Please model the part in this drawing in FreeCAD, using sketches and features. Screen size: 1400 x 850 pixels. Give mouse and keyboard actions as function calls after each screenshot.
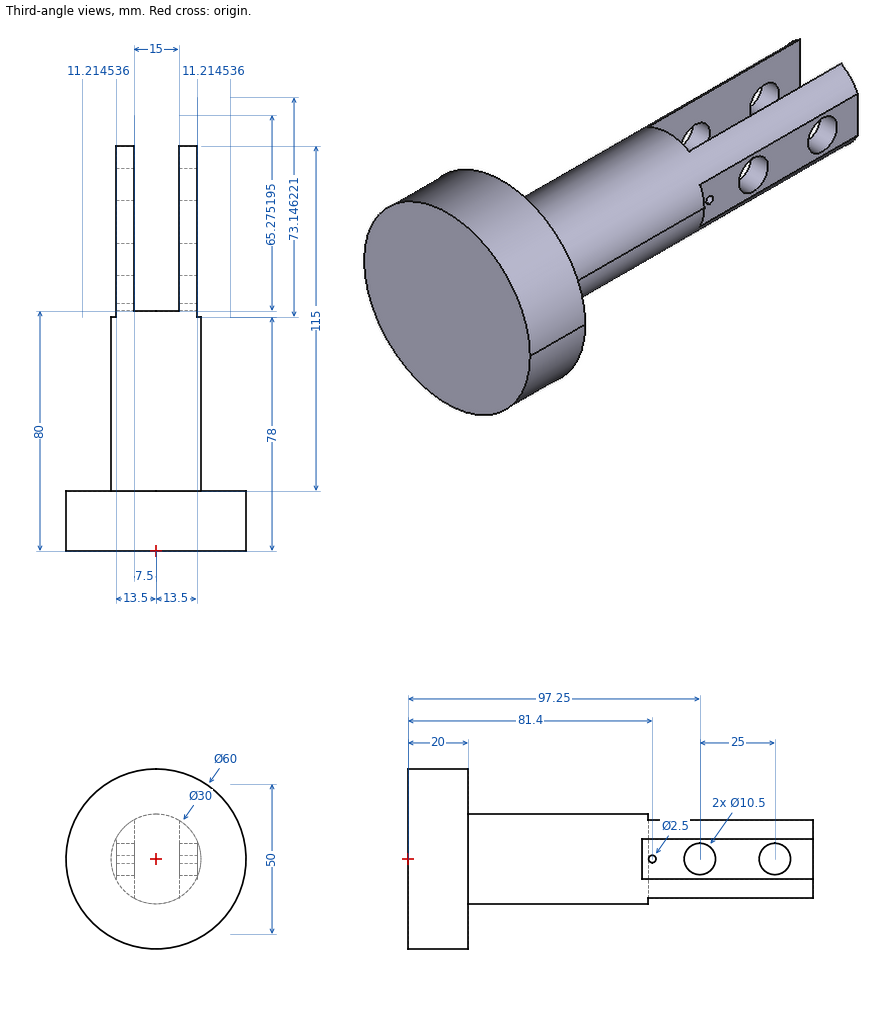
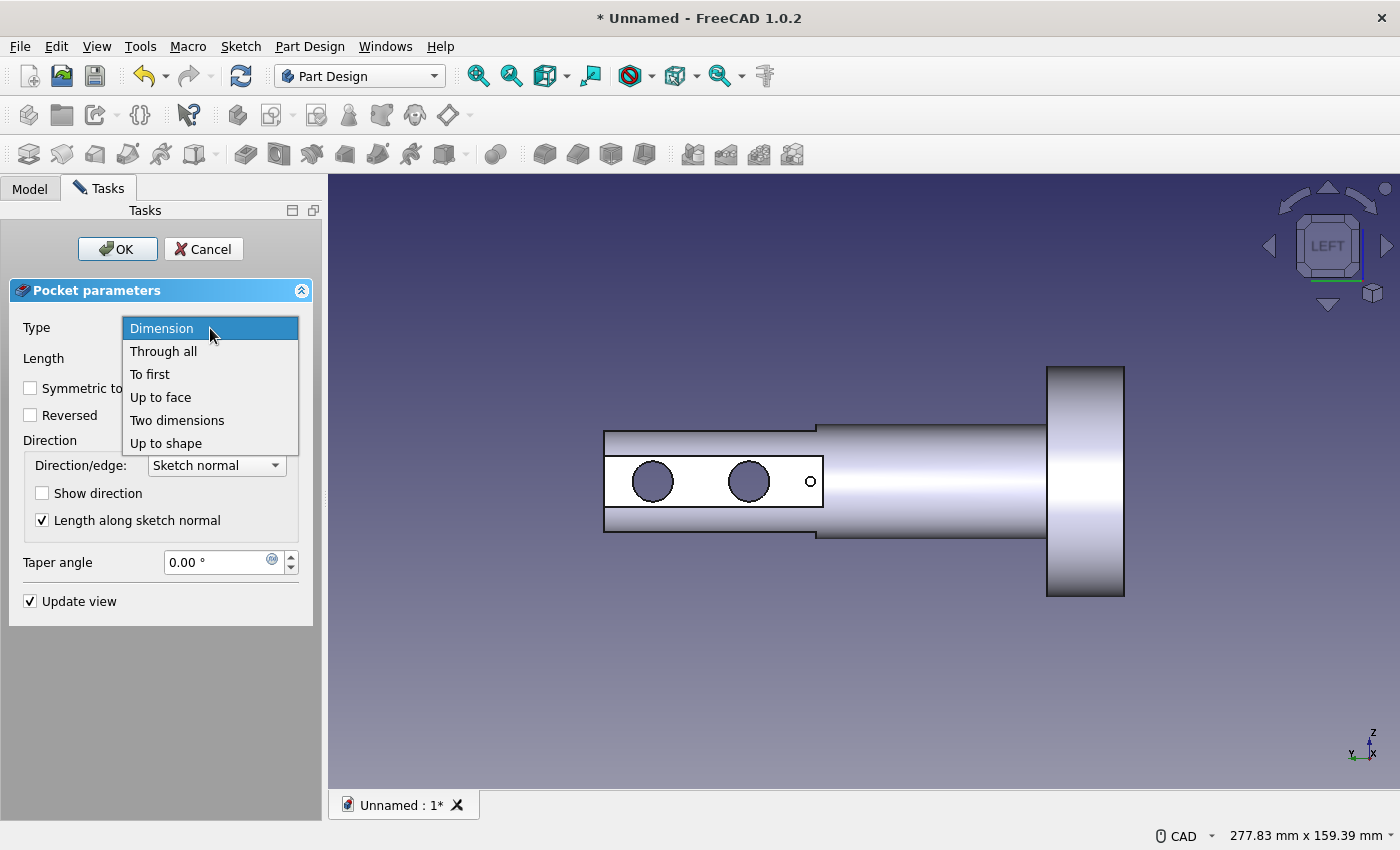
click(208, 352)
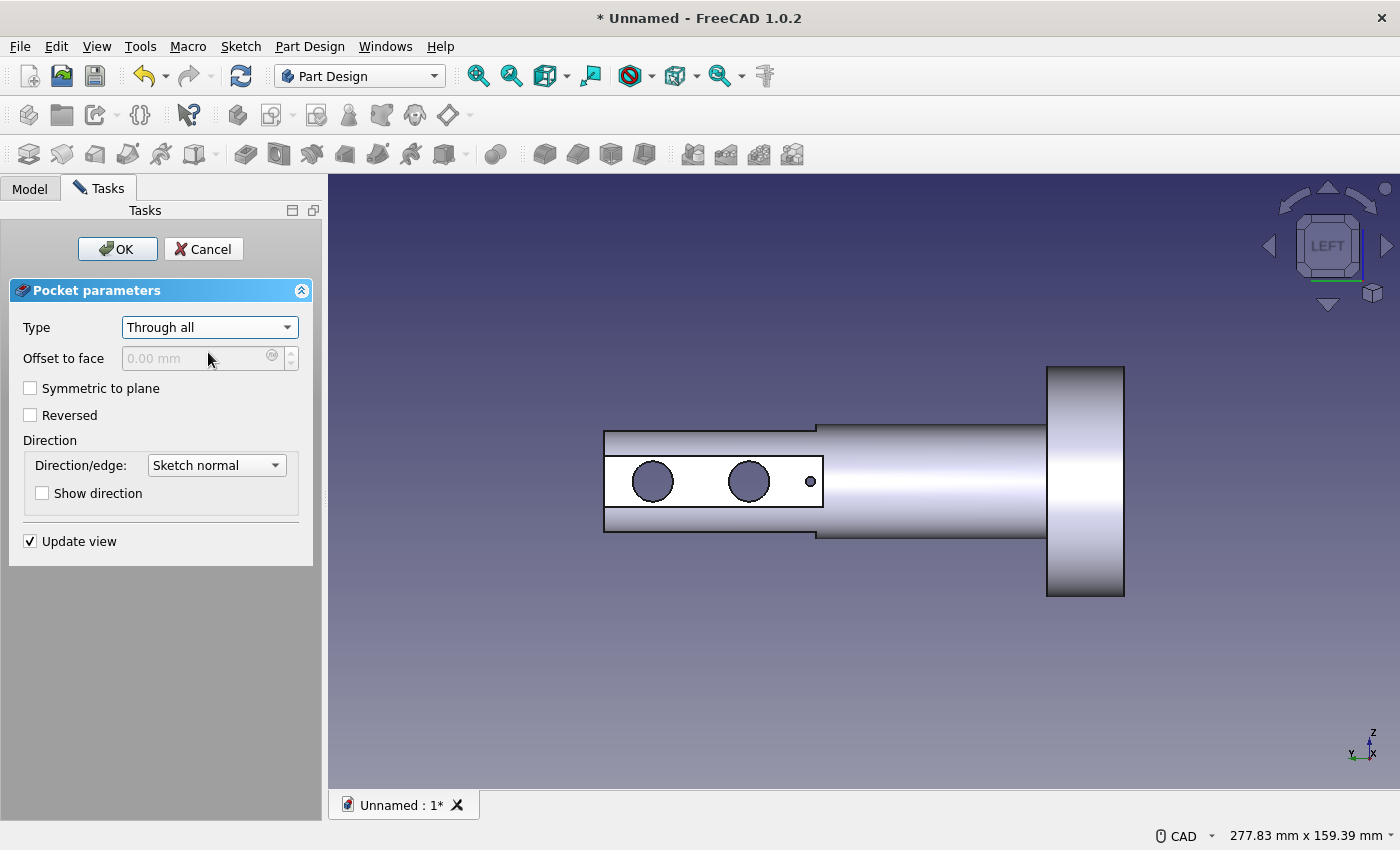
click(118, 249)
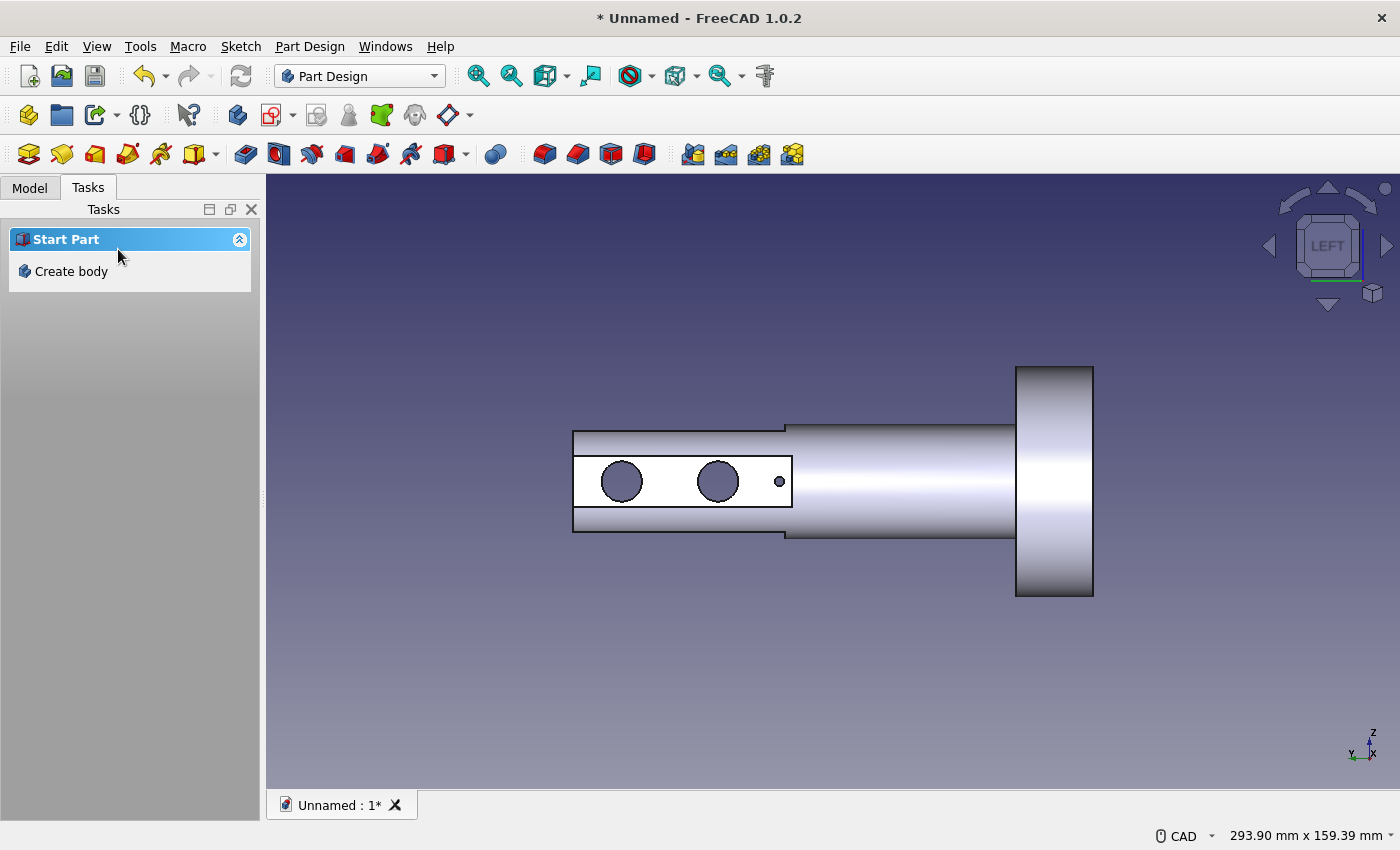
key(0)